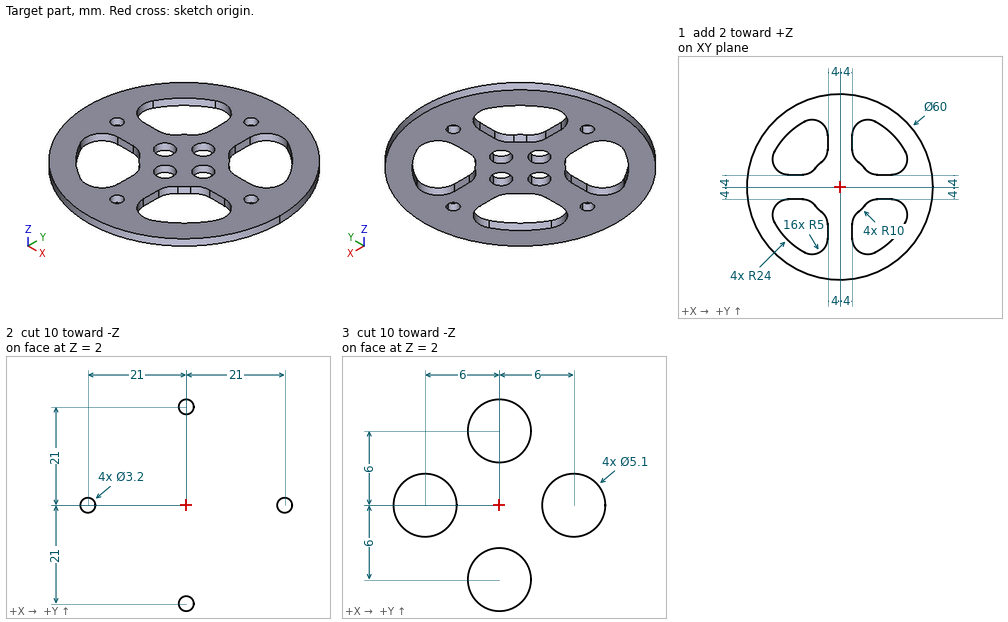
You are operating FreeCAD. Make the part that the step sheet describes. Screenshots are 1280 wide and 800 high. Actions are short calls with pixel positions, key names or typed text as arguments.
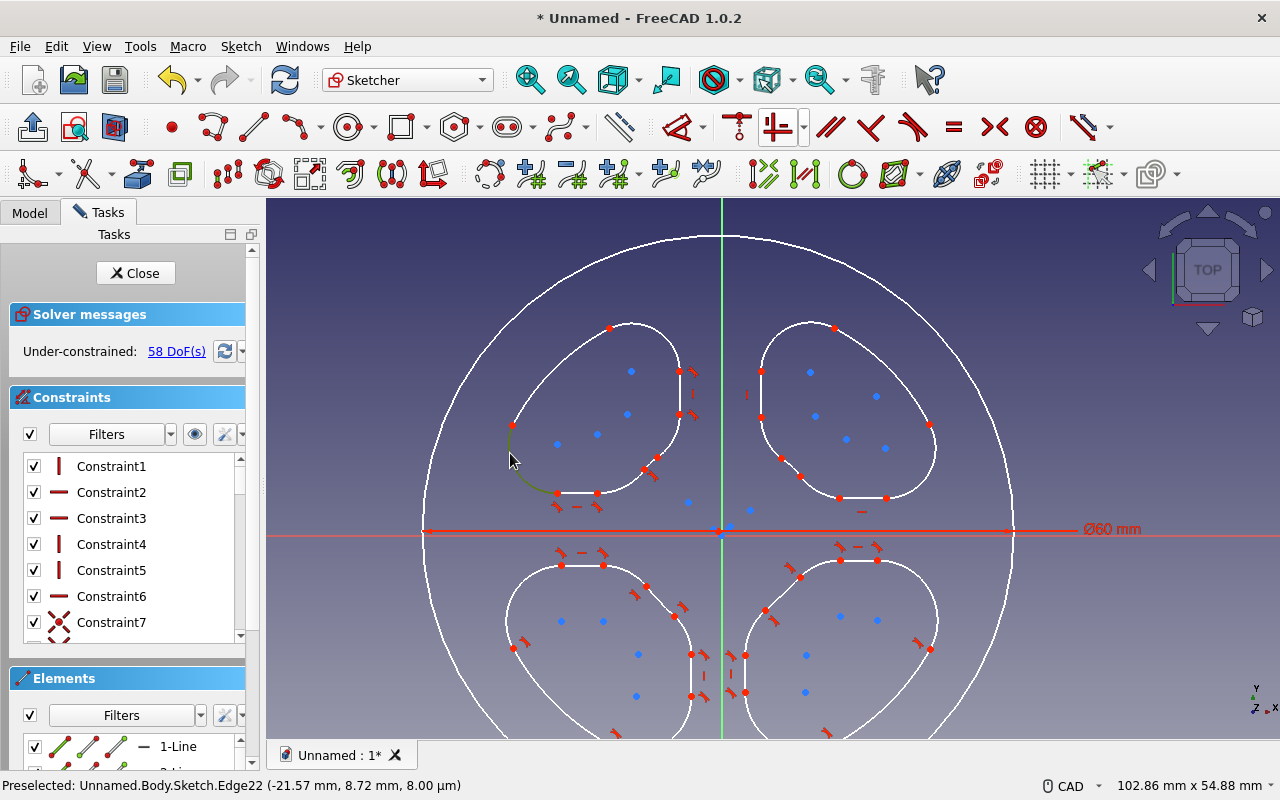
click(575, 351)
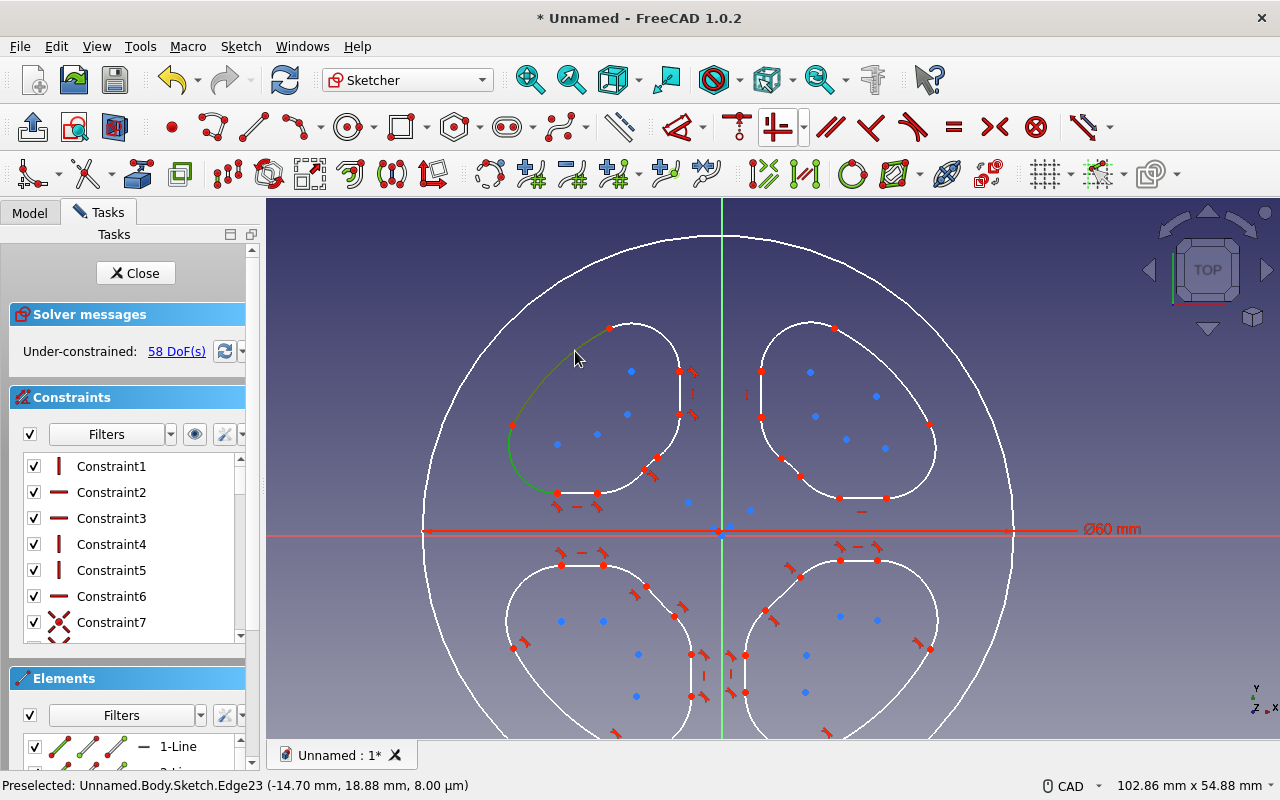
key(t)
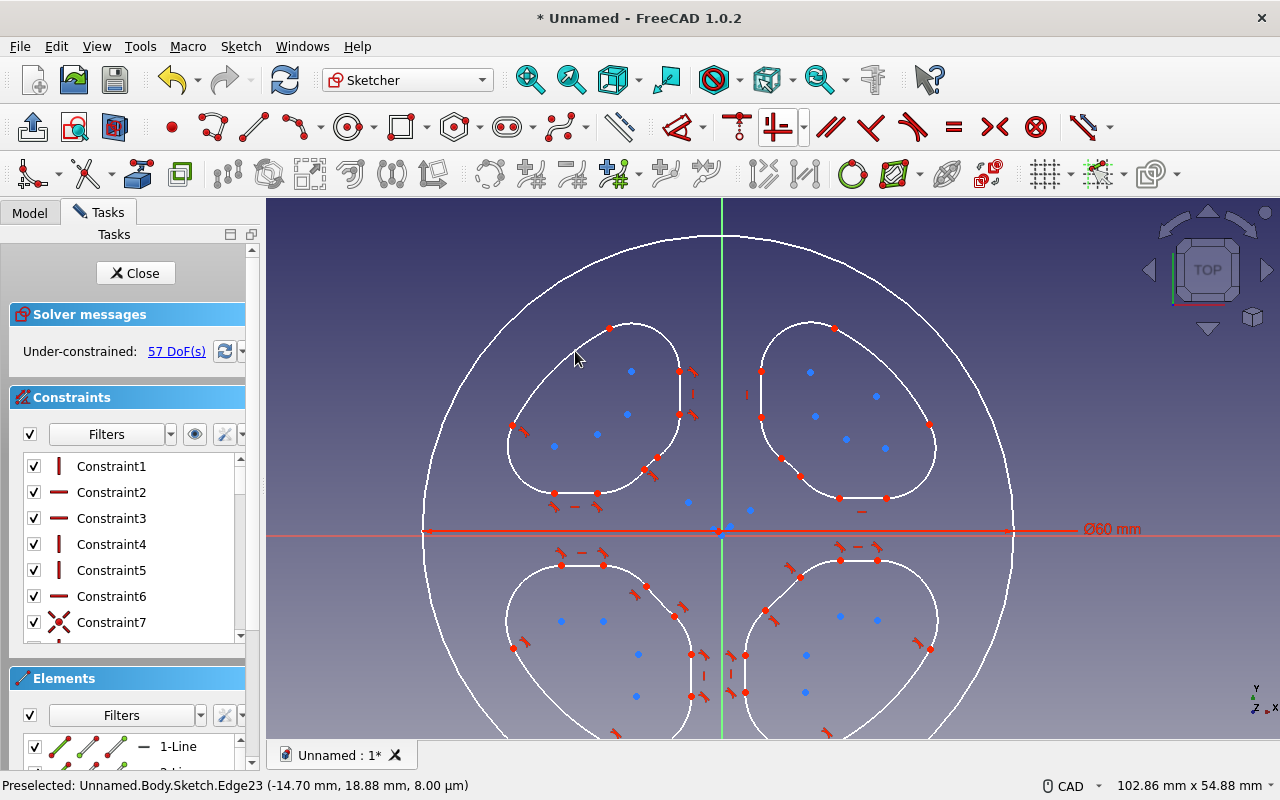
click(575, 351)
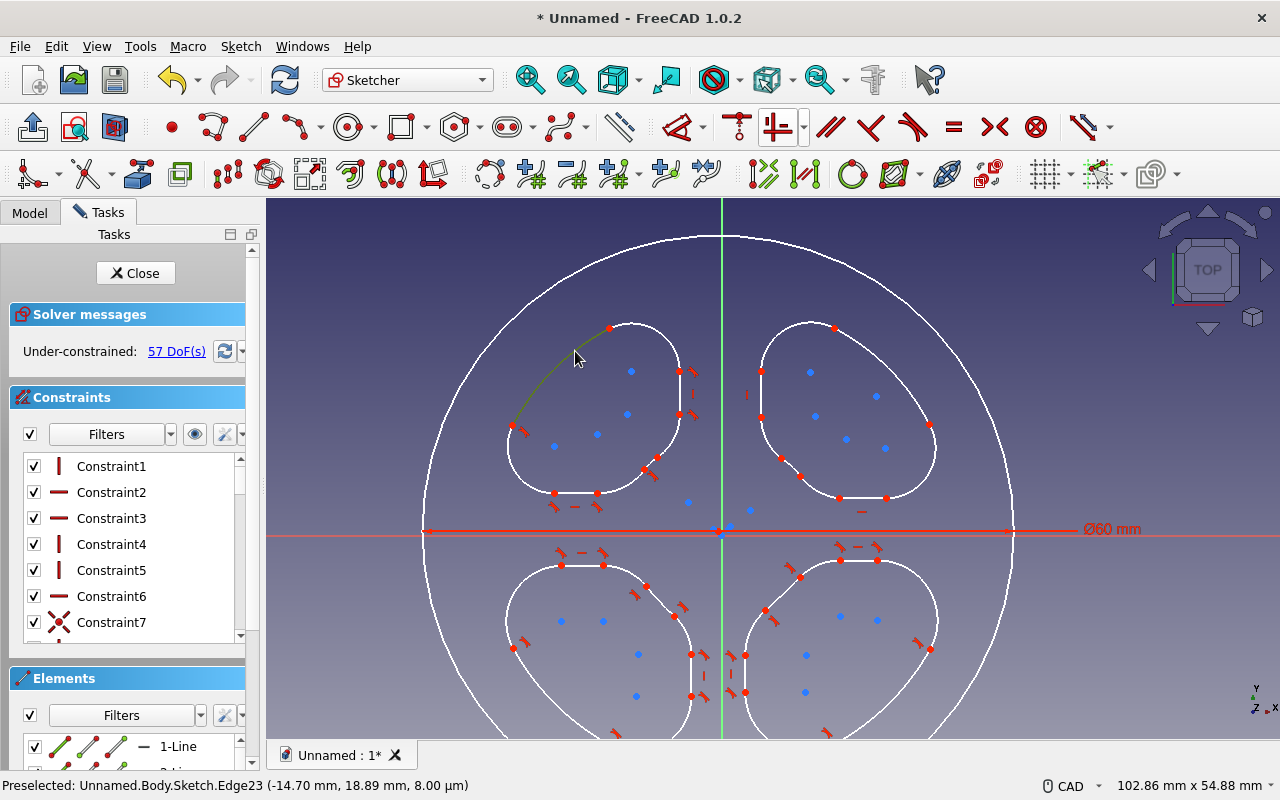
click(671, 344)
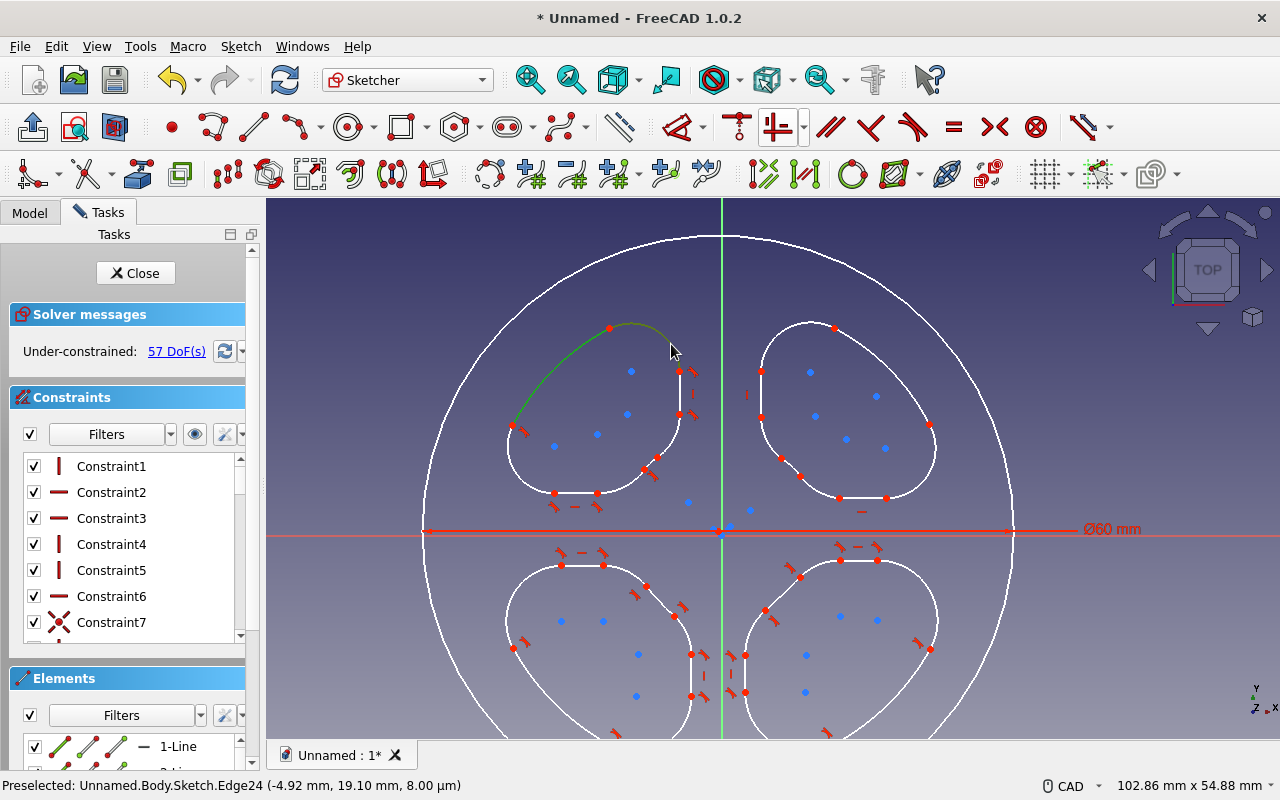
key(t)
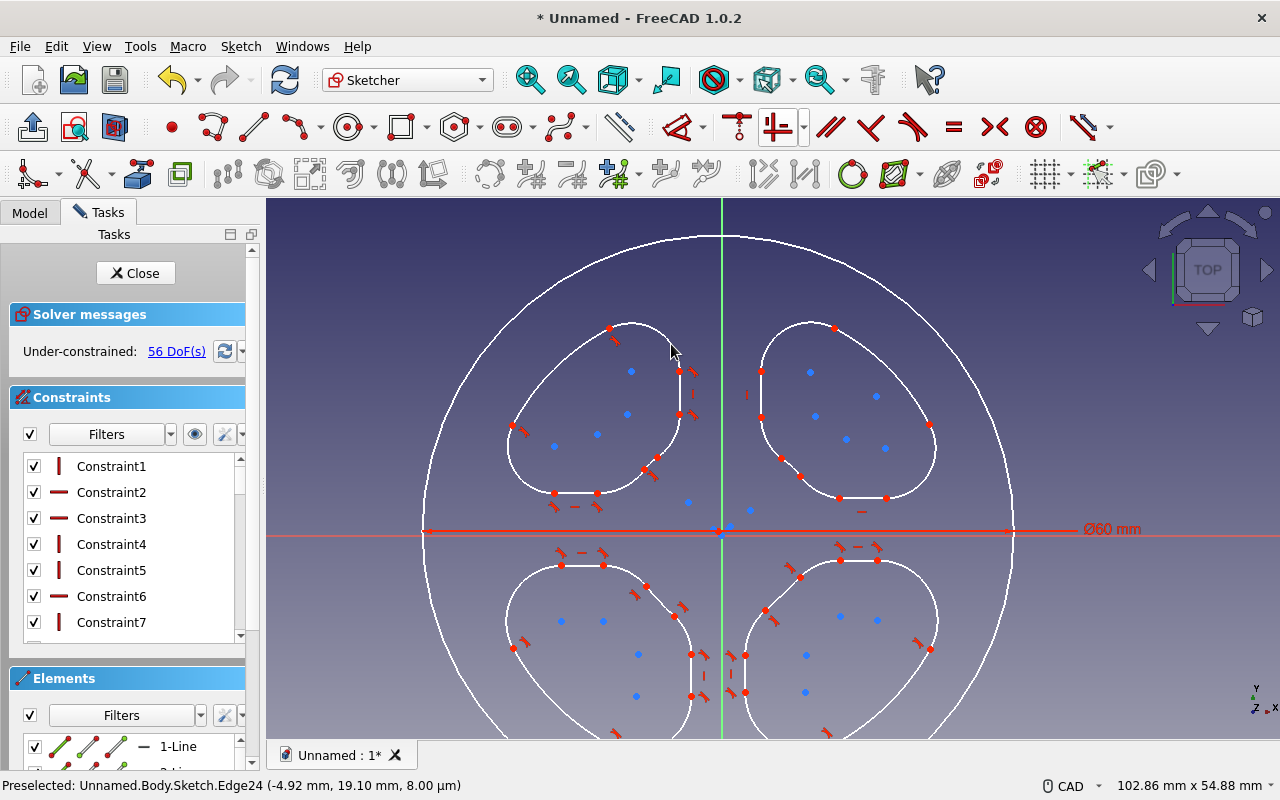
click(761, 404)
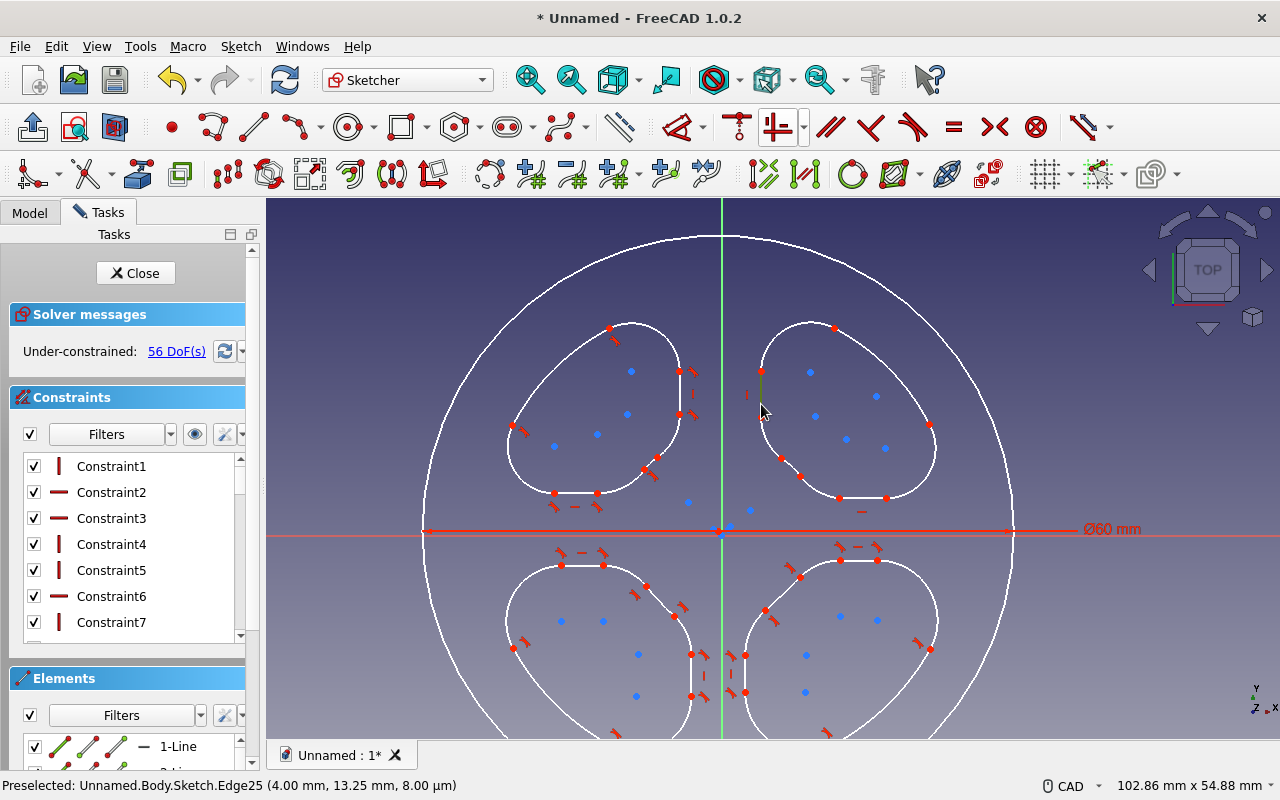
click(805, 323)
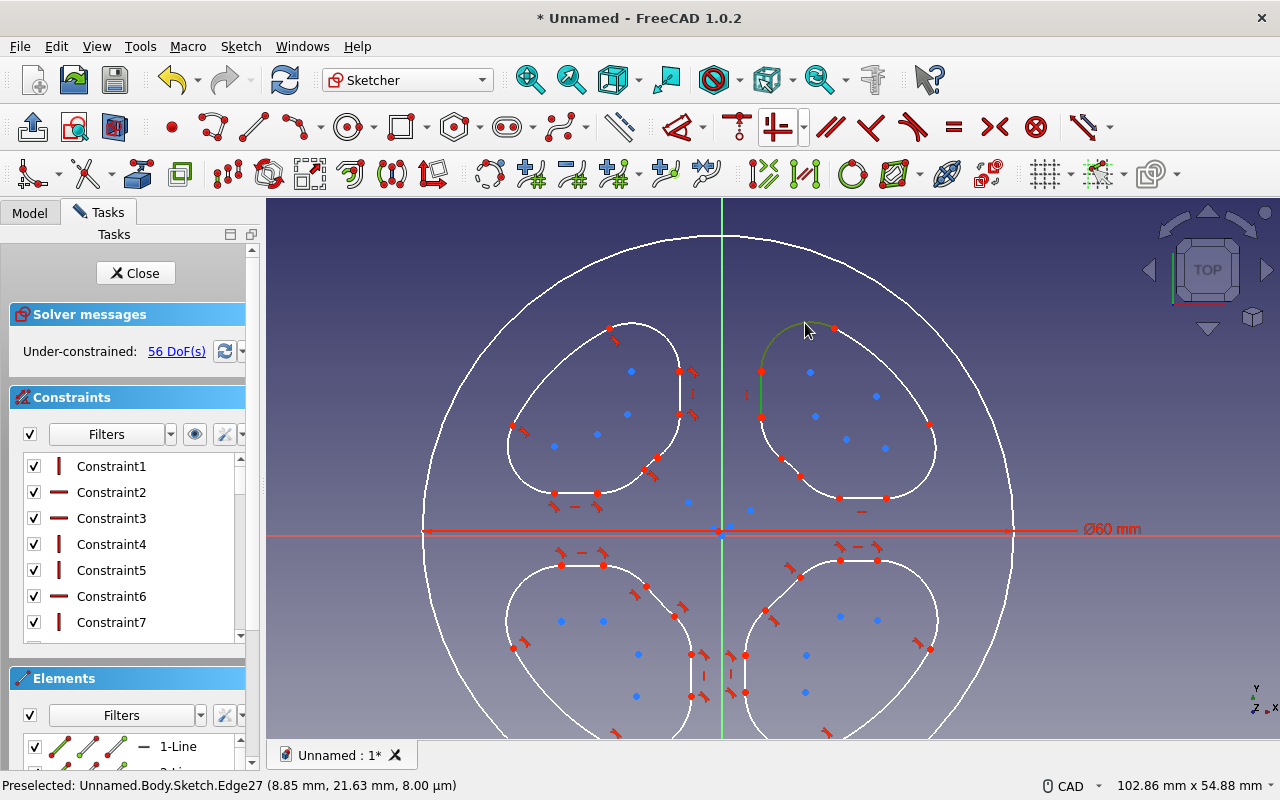
key(t)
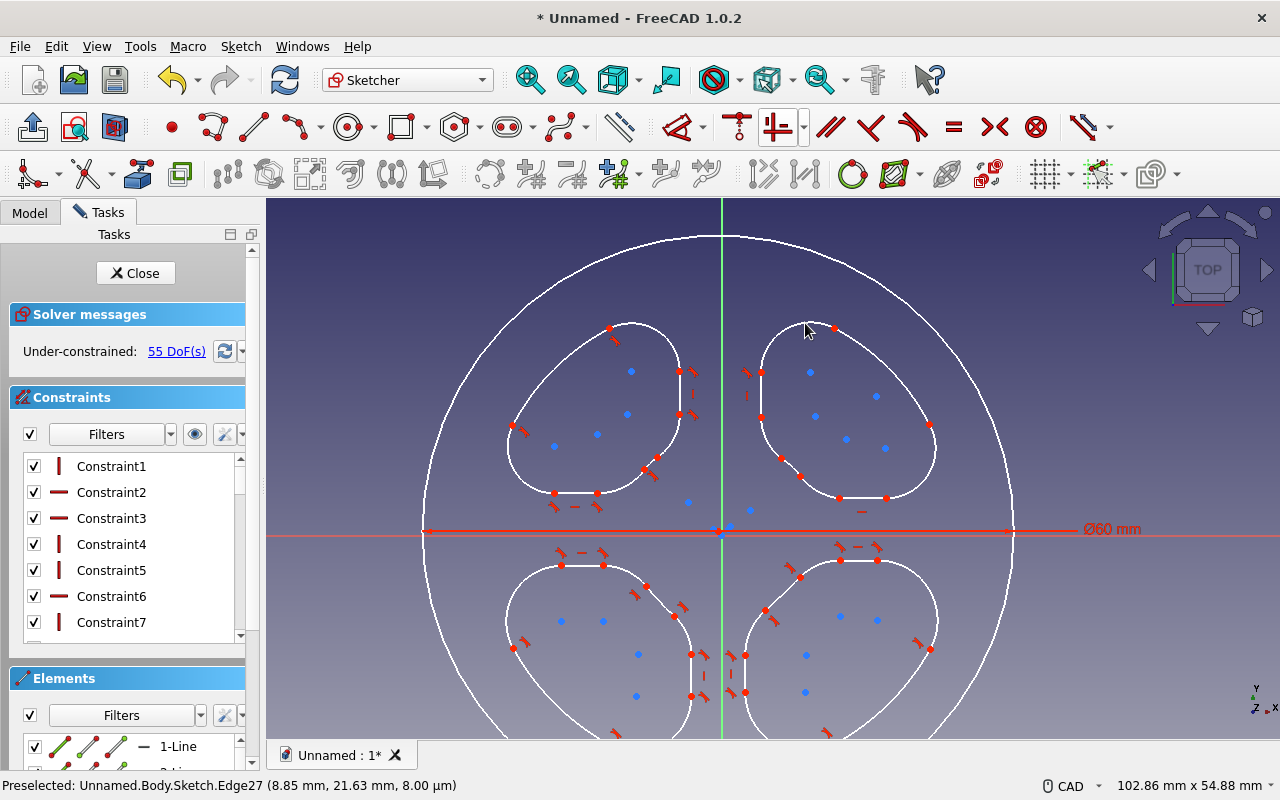
click(761, 404)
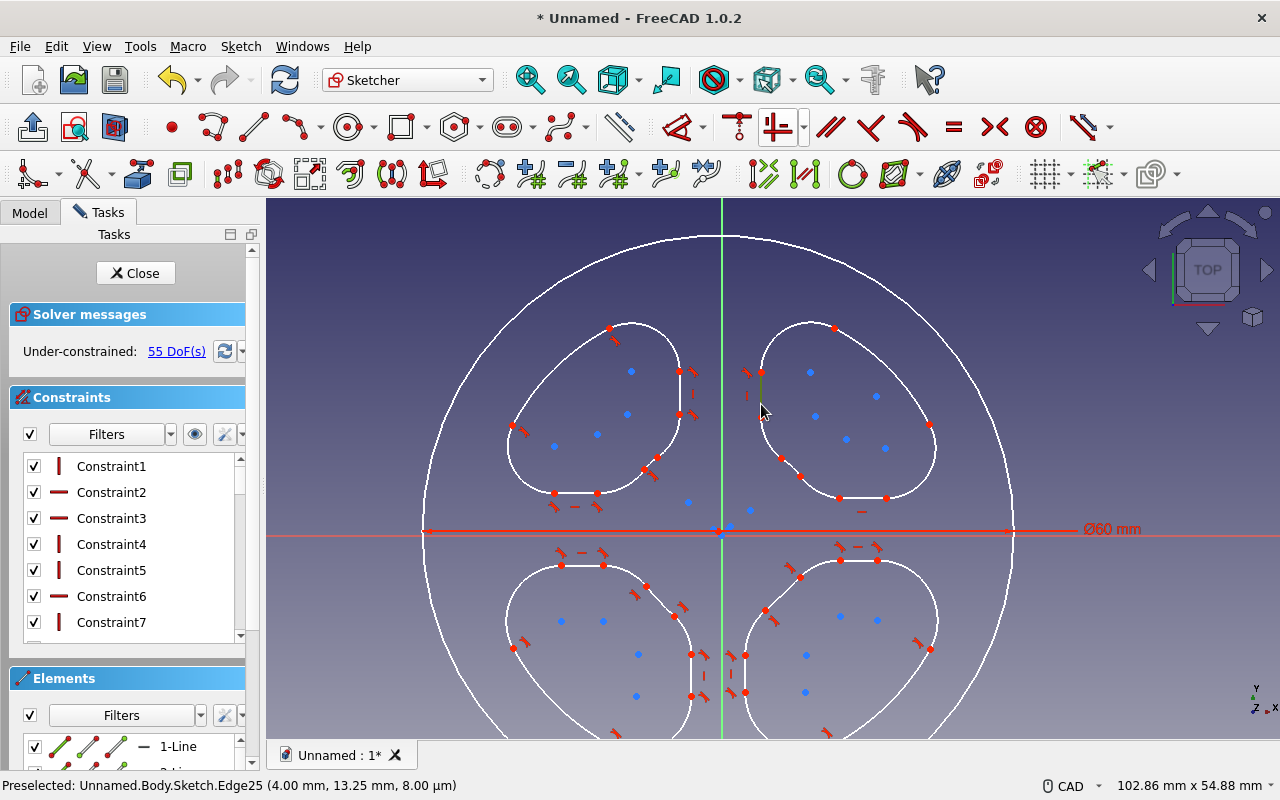
click(763, 432)